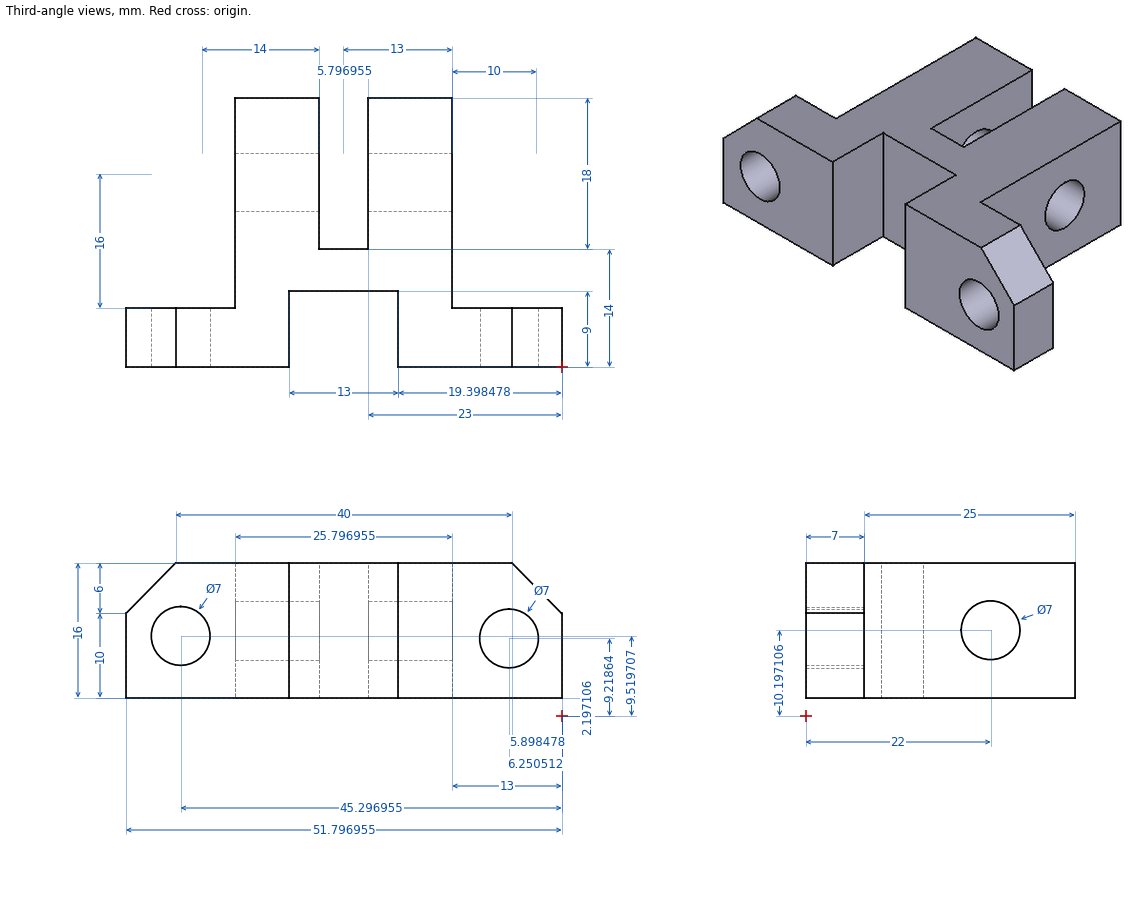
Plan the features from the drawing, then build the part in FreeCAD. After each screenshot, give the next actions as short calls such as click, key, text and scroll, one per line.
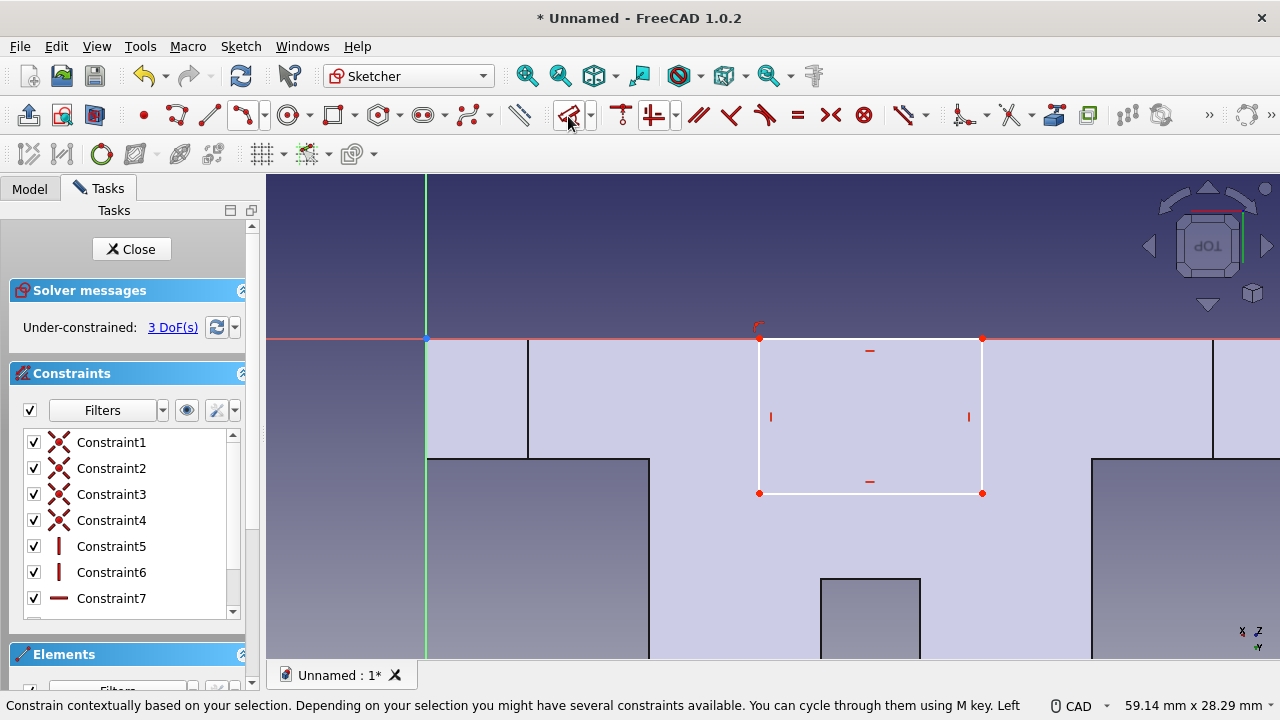
click(759, 385)
click(793, 416)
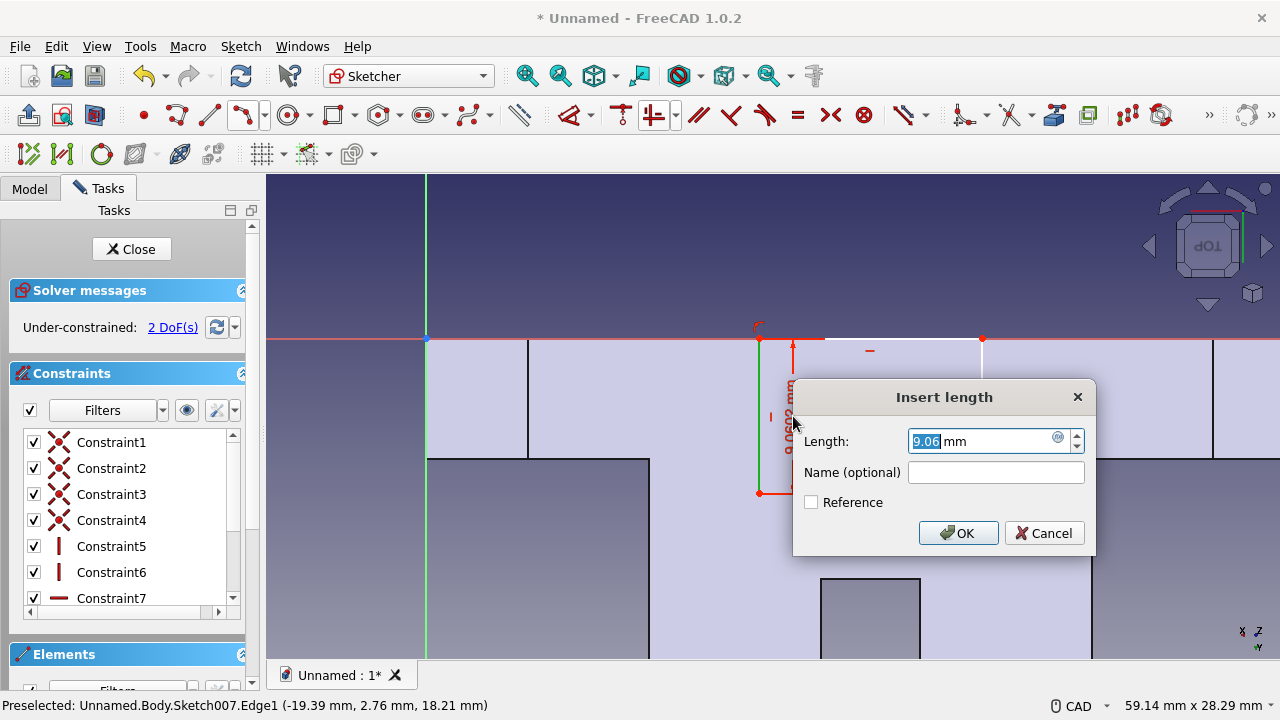
text(9)
key(Return)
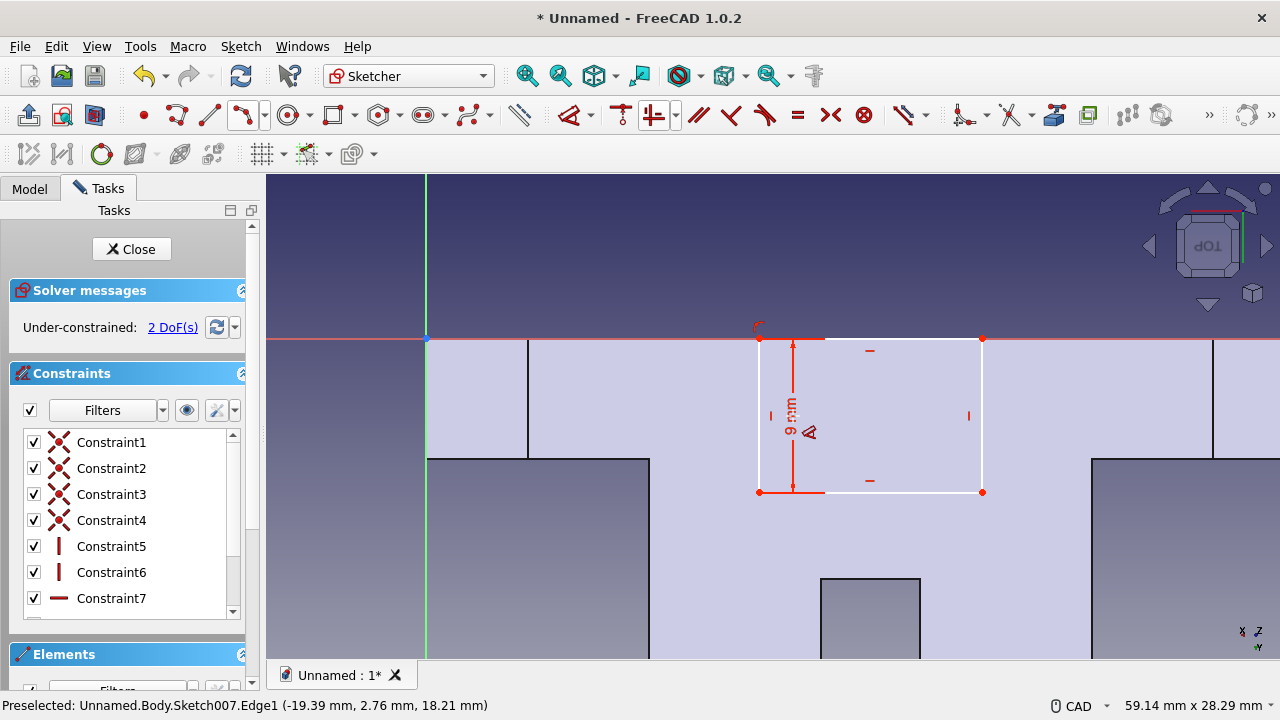
click(826, 493)
click(871, 527)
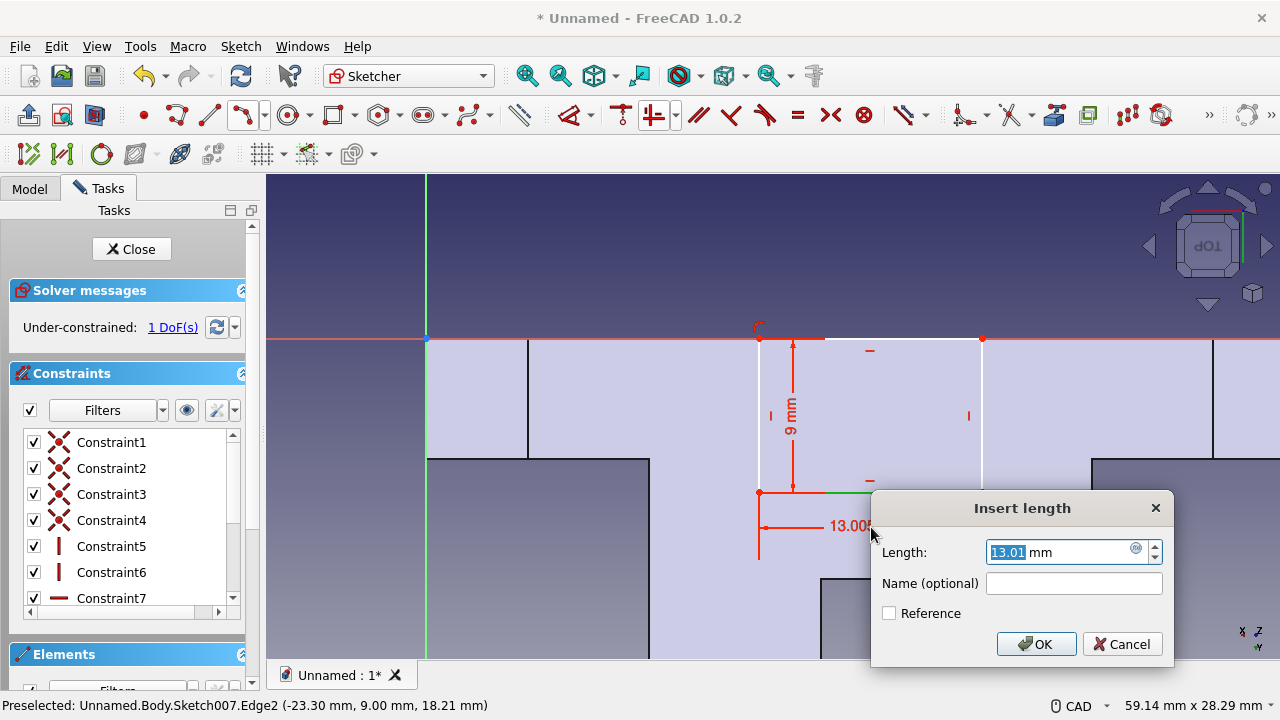
text(13)
key(Return)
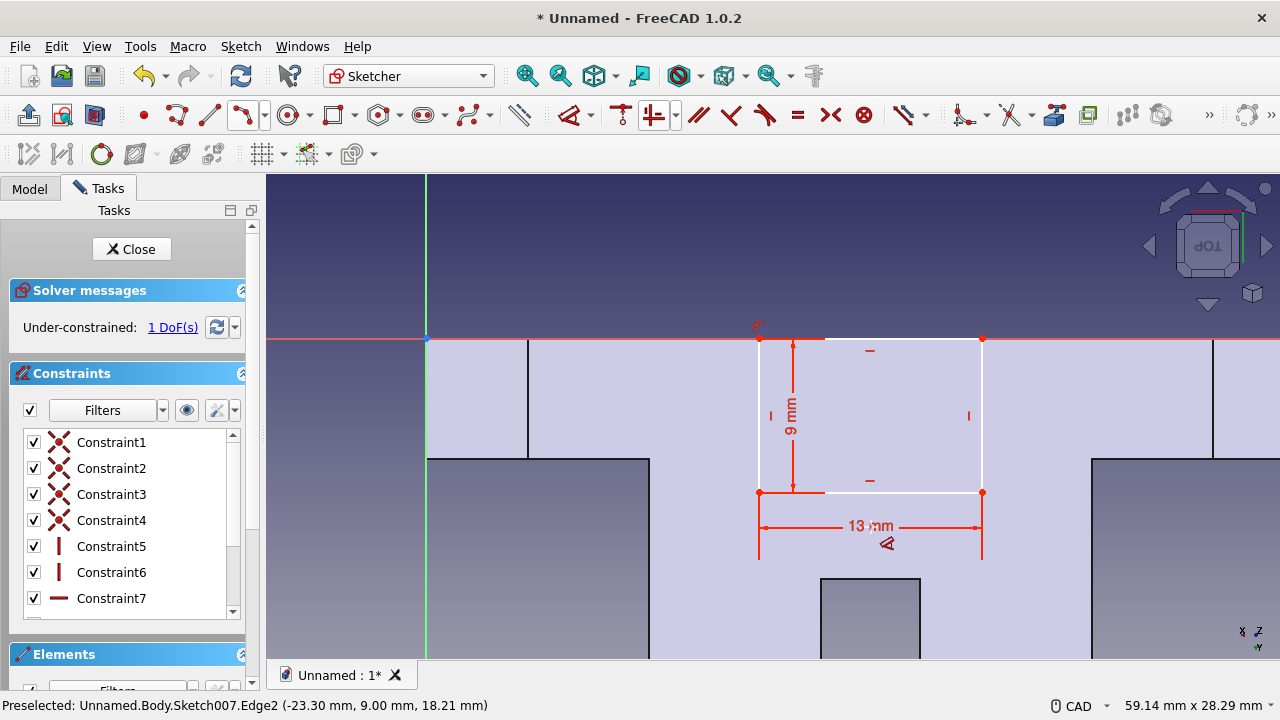
click(759, 339)
click(593, 305)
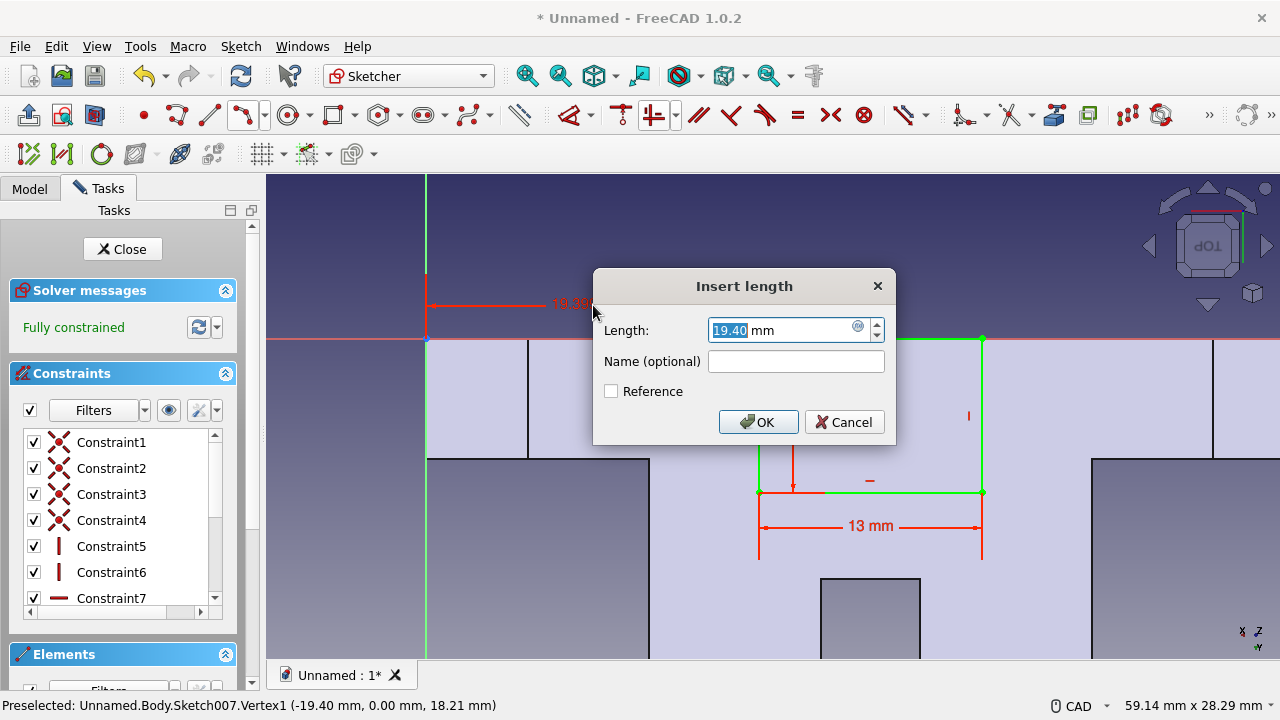
text(19.398478)
key(Return)
key(Escape)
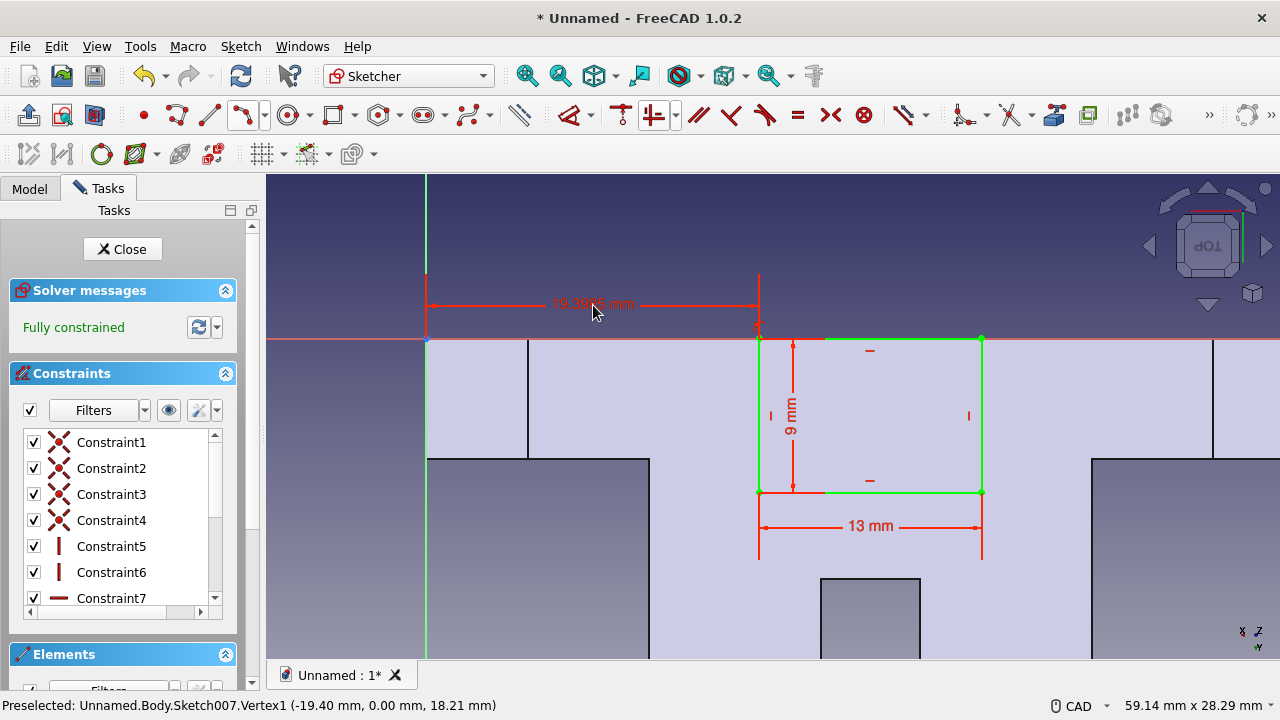
click(123, 249)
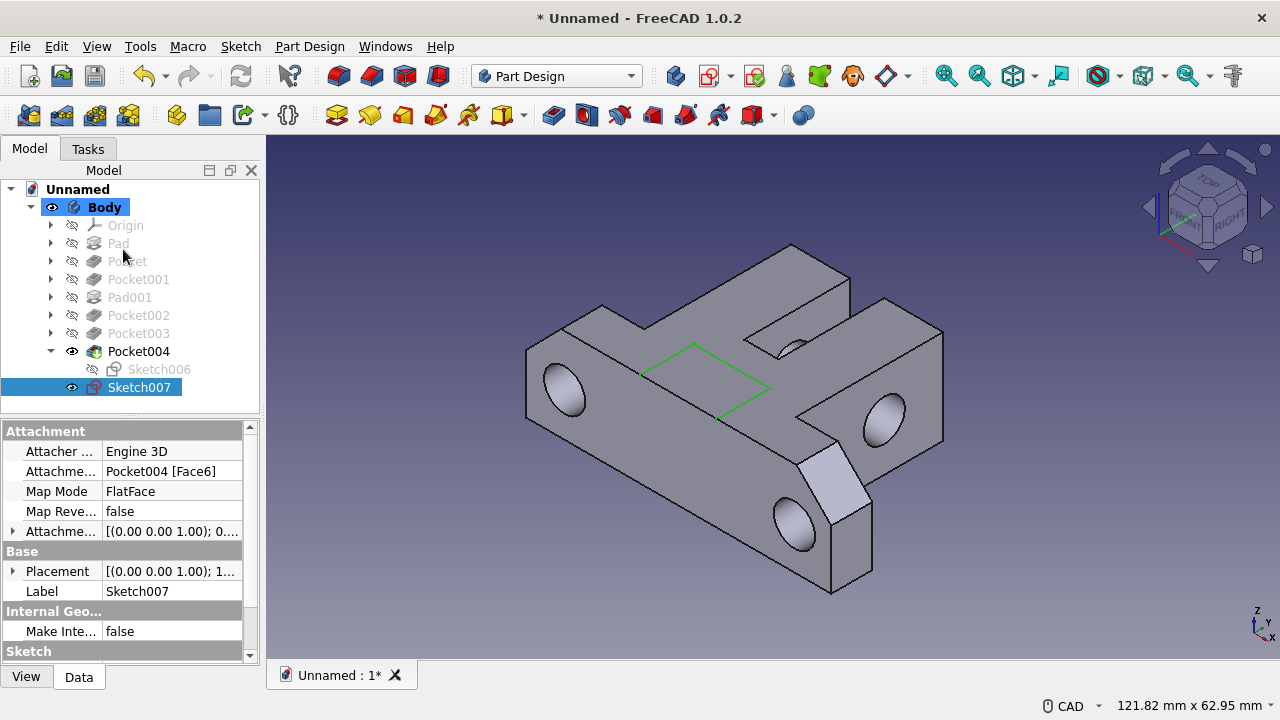
click(554, 116)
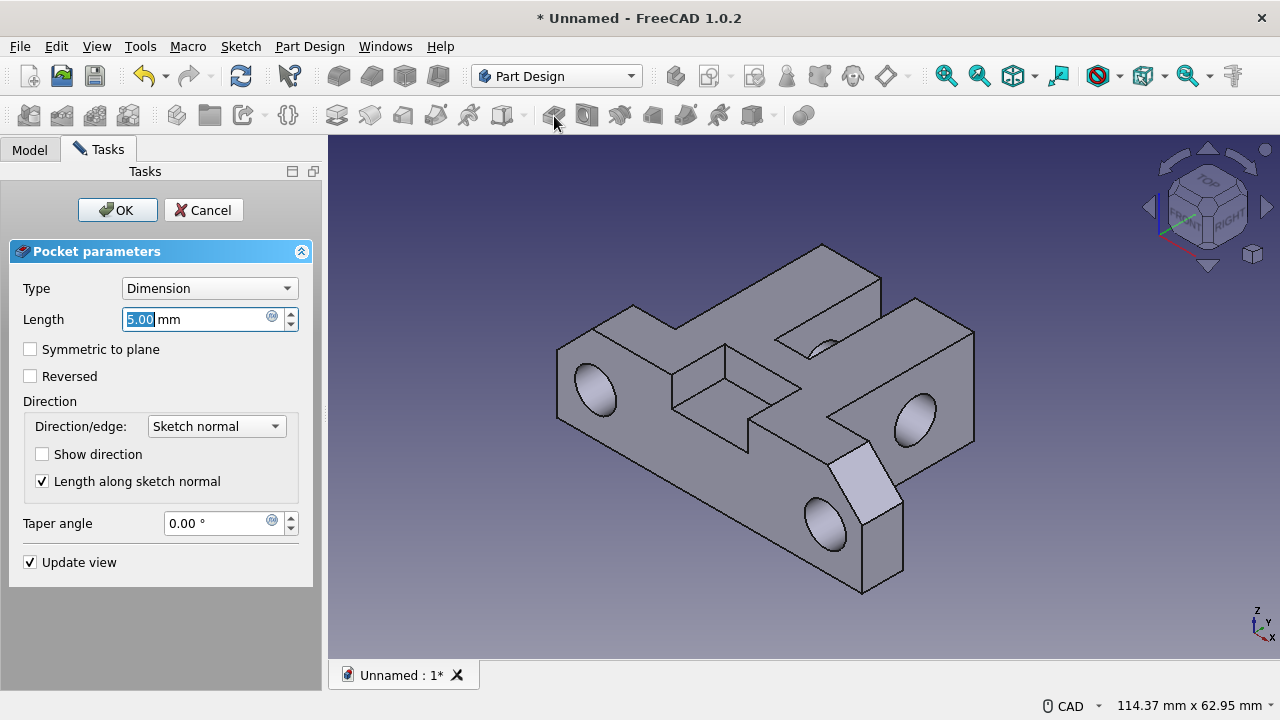
click(210, 288)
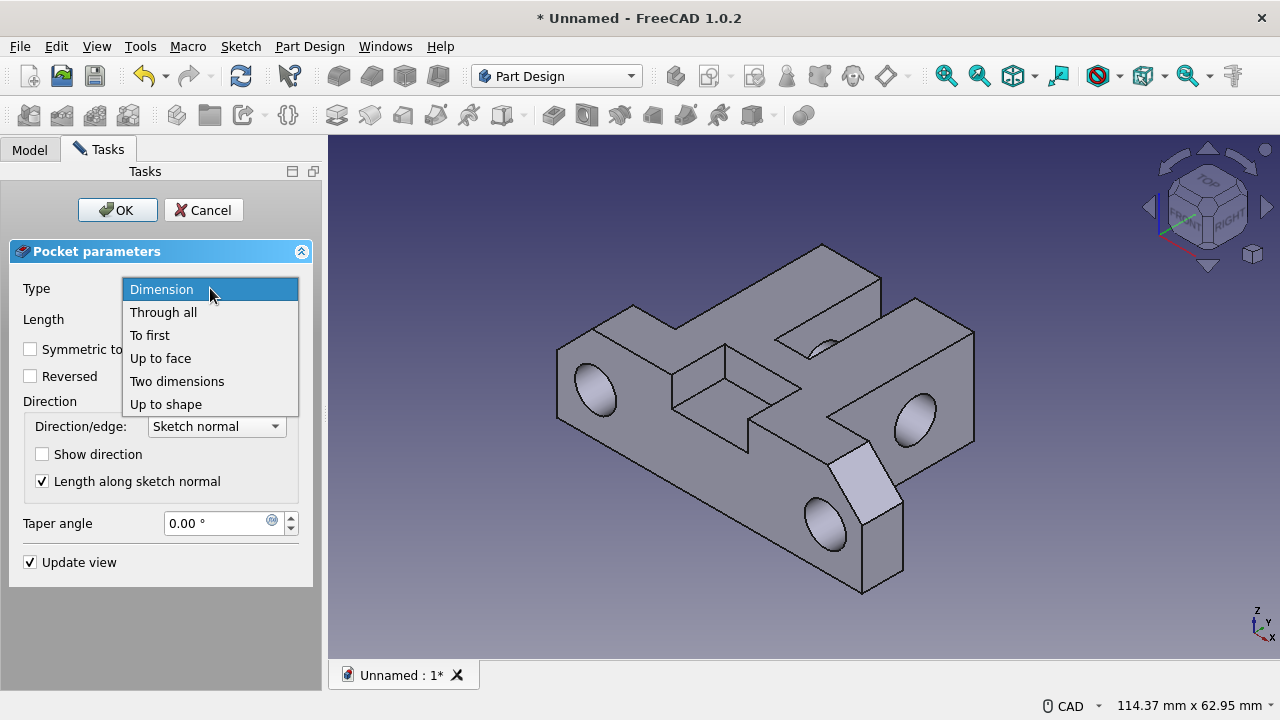
click(208, 382)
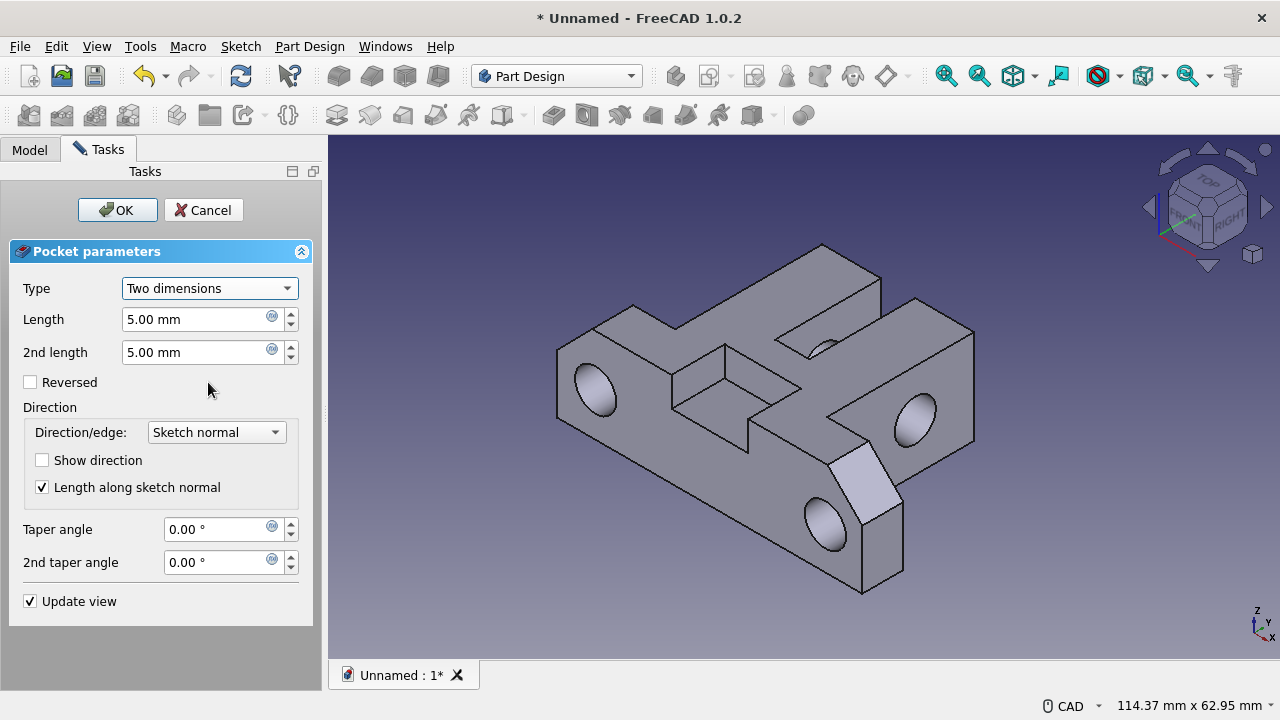
triple_click(204, 320)